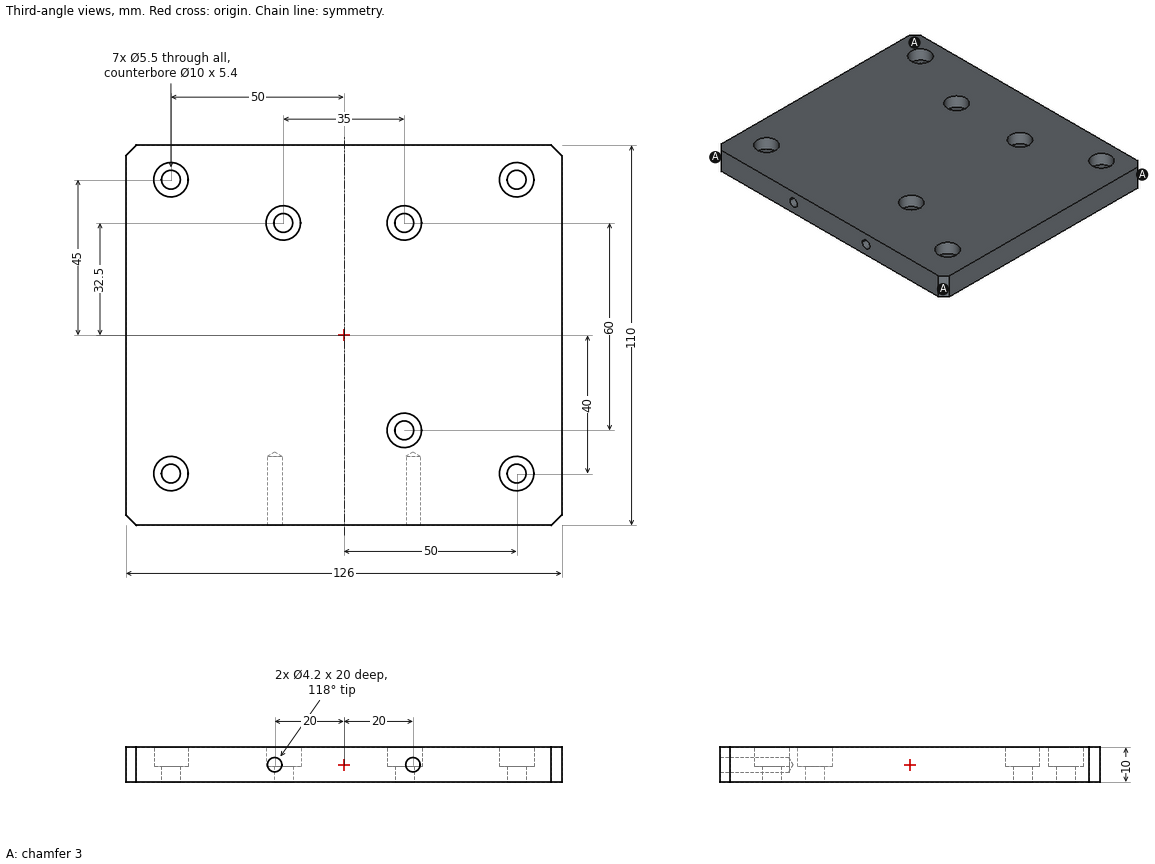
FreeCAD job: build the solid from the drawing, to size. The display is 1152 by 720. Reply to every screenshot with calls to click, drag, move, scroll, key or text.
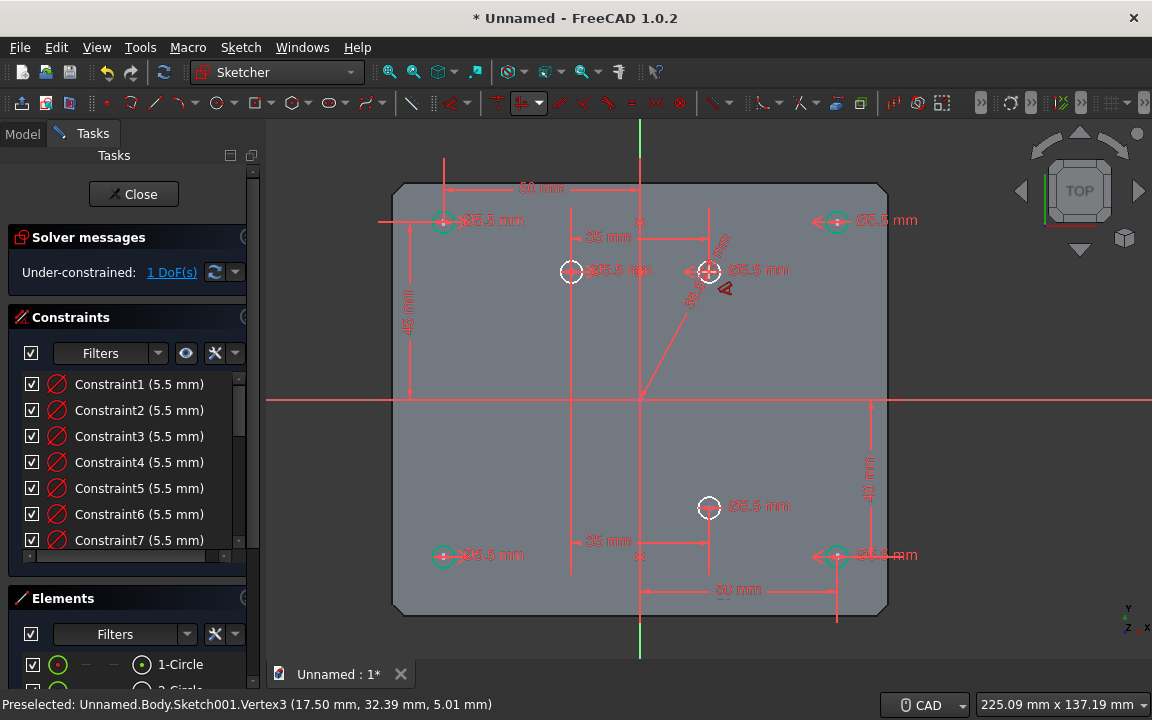
click(709, 508)
click(743, 336)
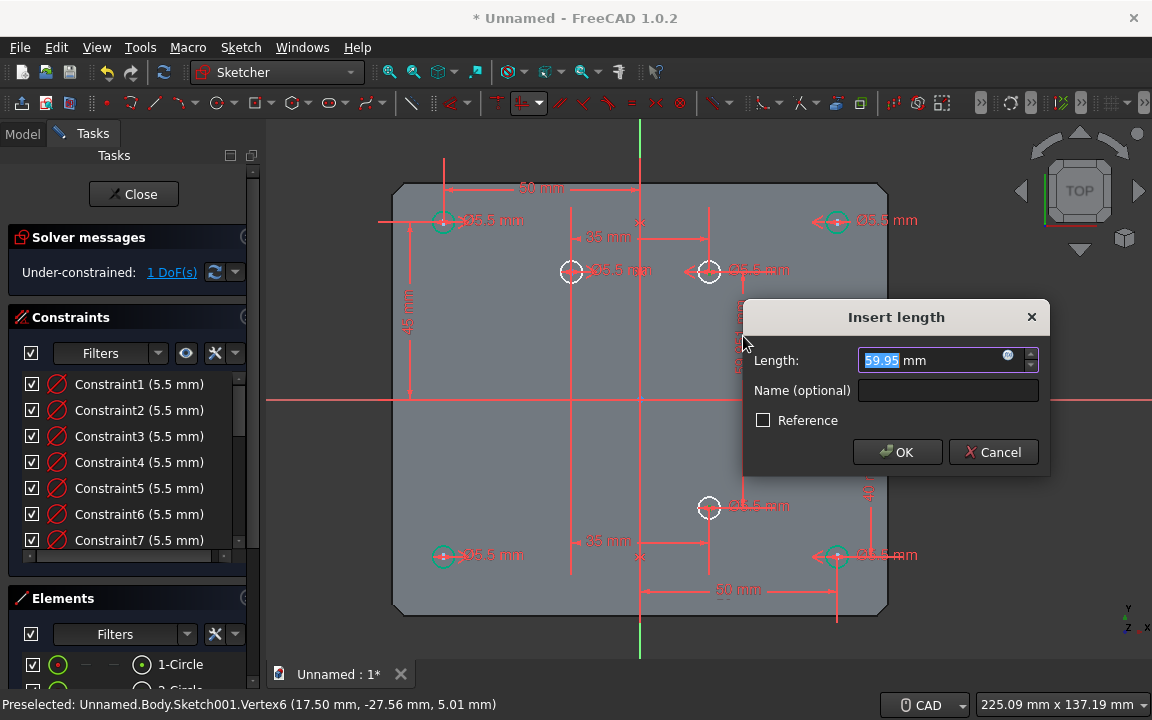
text(60)
key(Return)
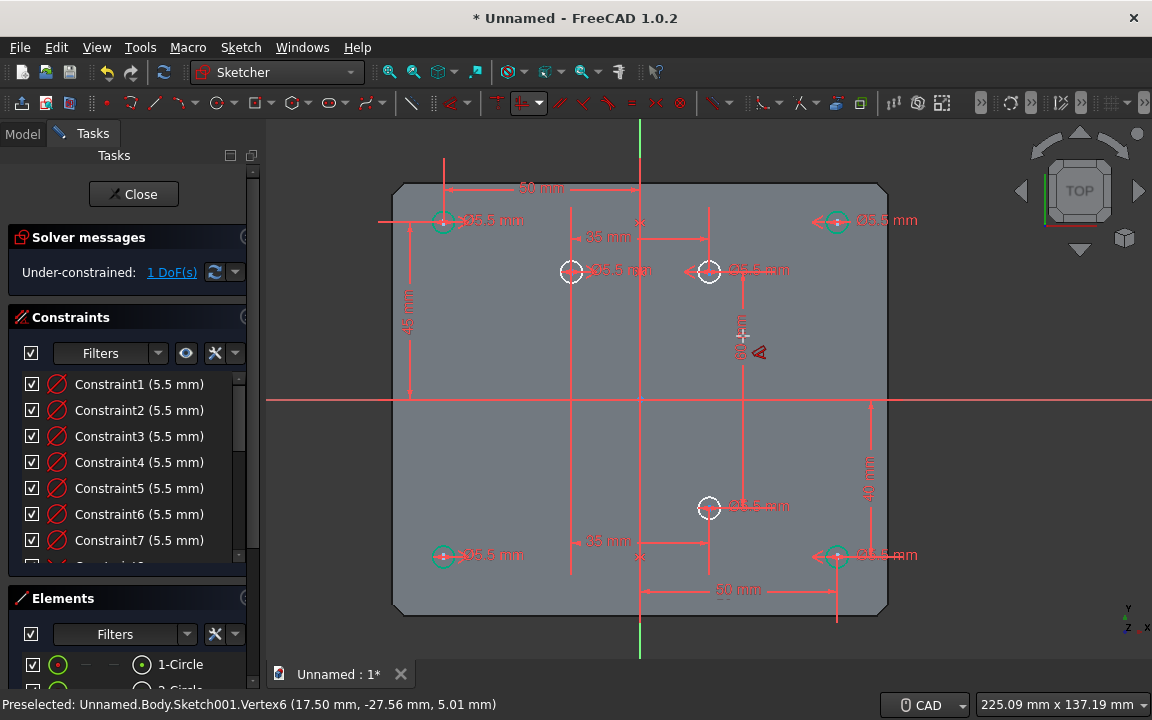
click(571, 272)
click(537, 336)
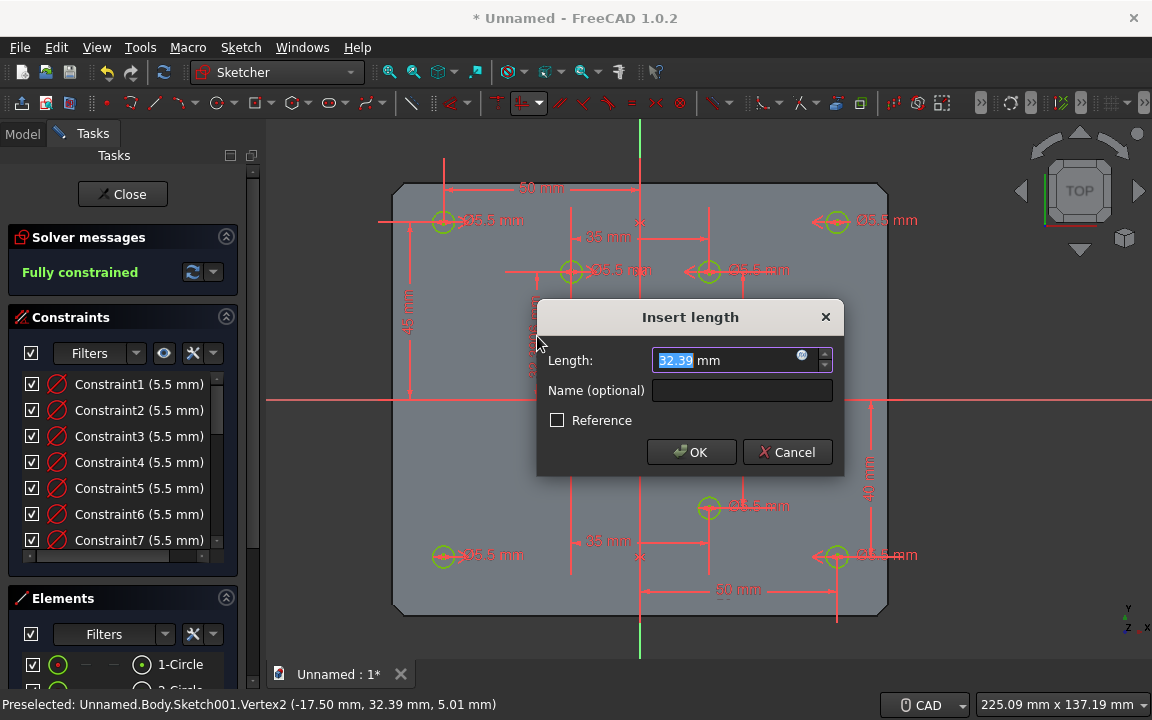
text(32.5)
key(Return)
key(Escape)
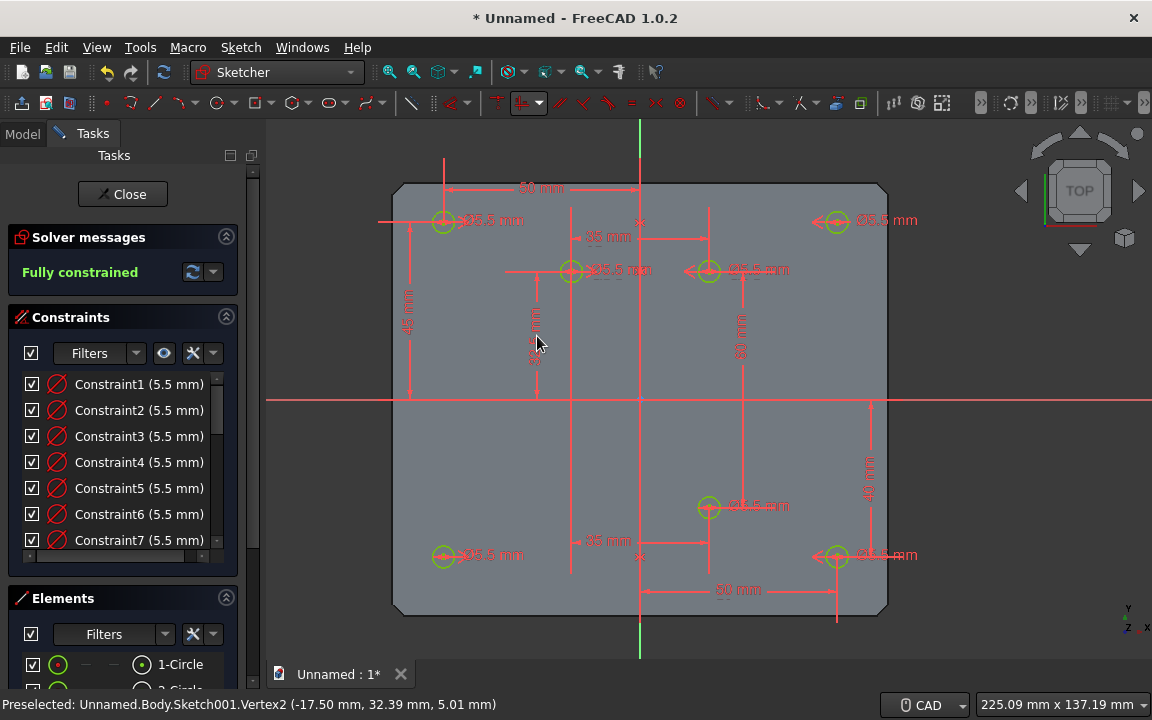
click(123, 194)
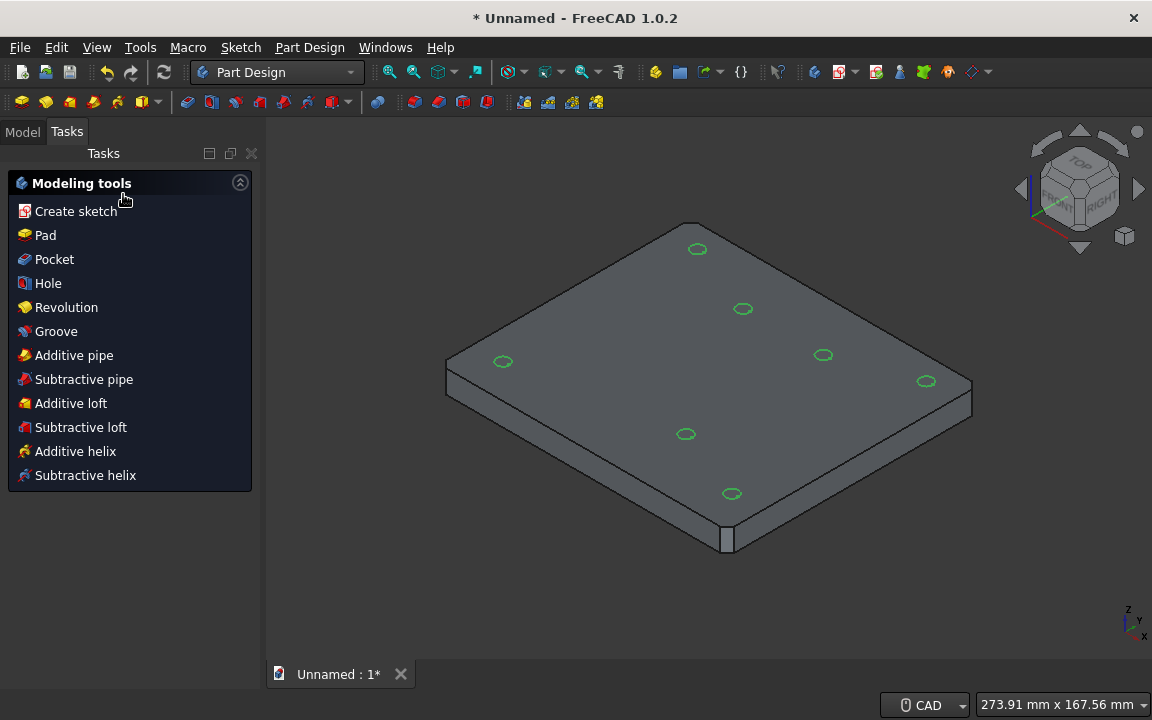
click(212, 102)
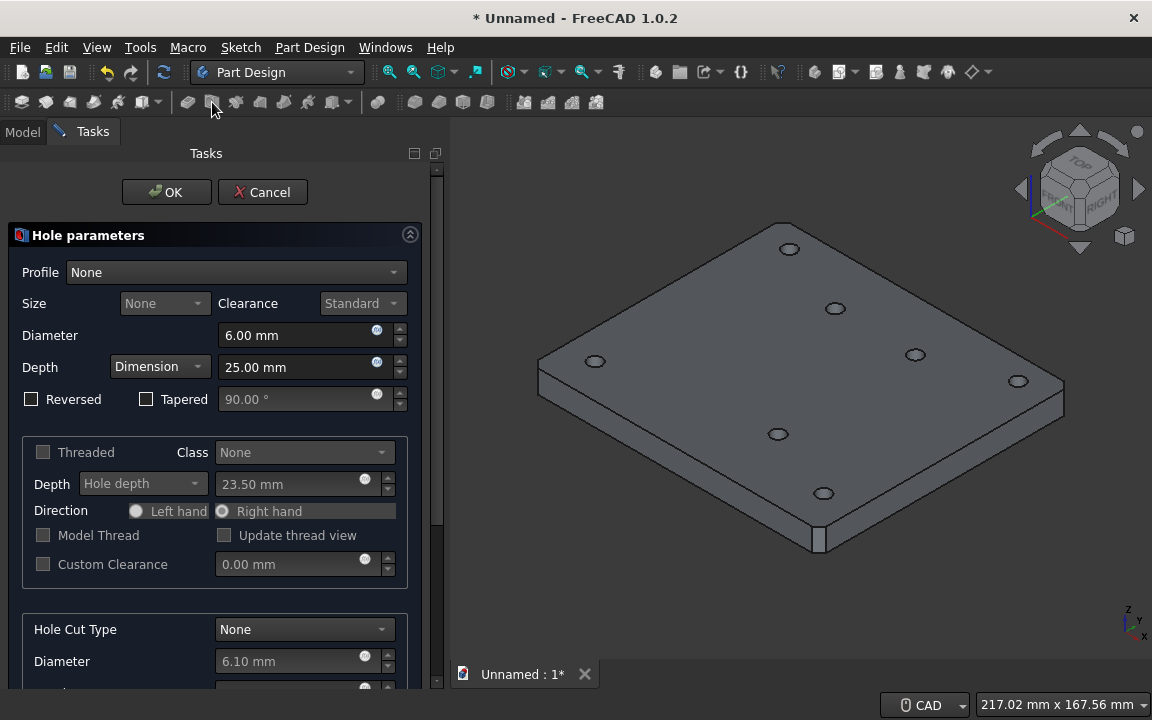
triple_click(305, 335)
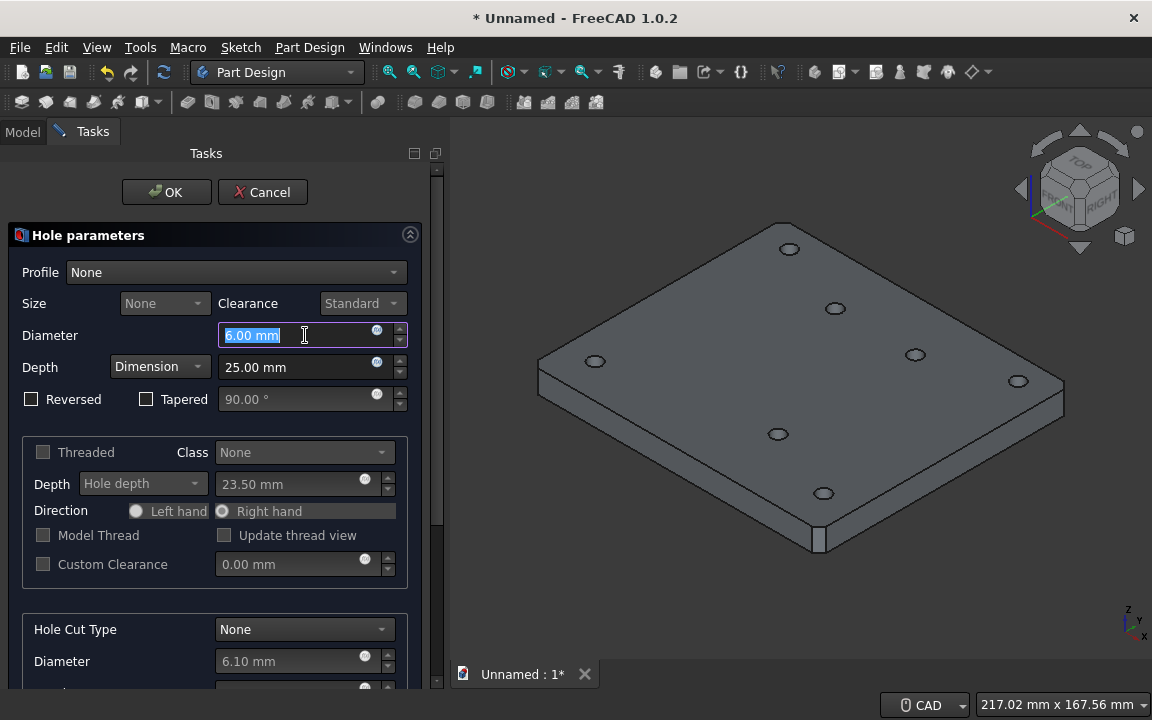
text(5.5)
key(Tab)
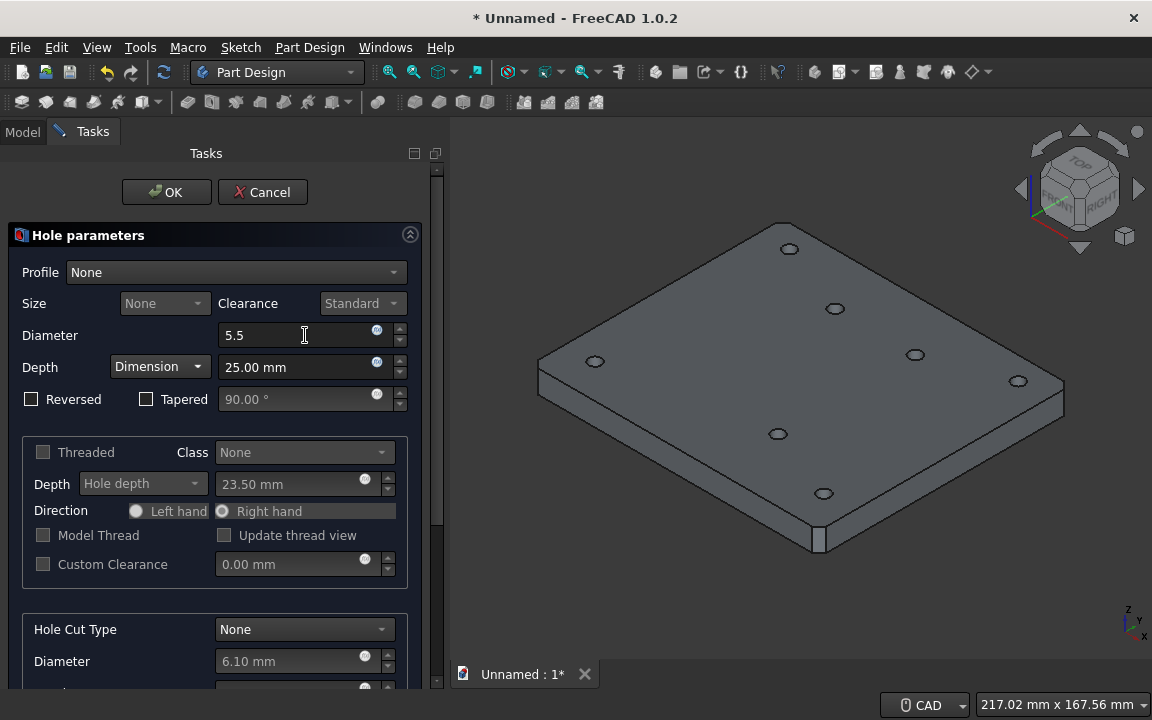
click(161, 366)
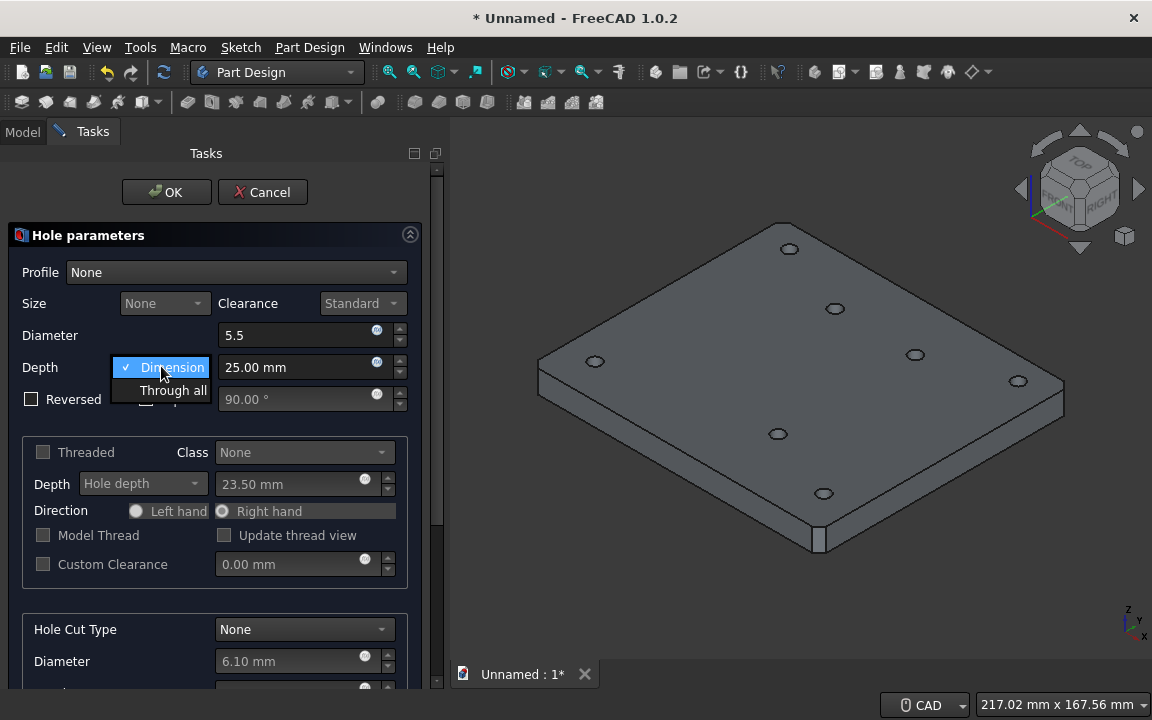
click(160, 390)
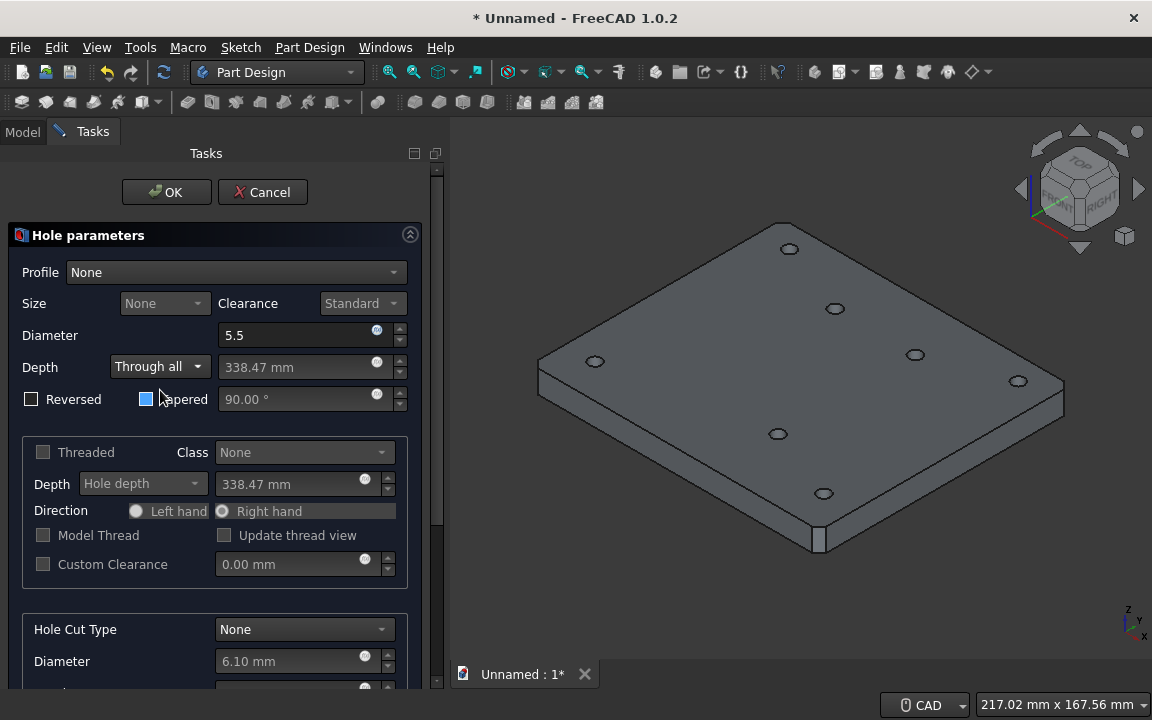
click(306, 630)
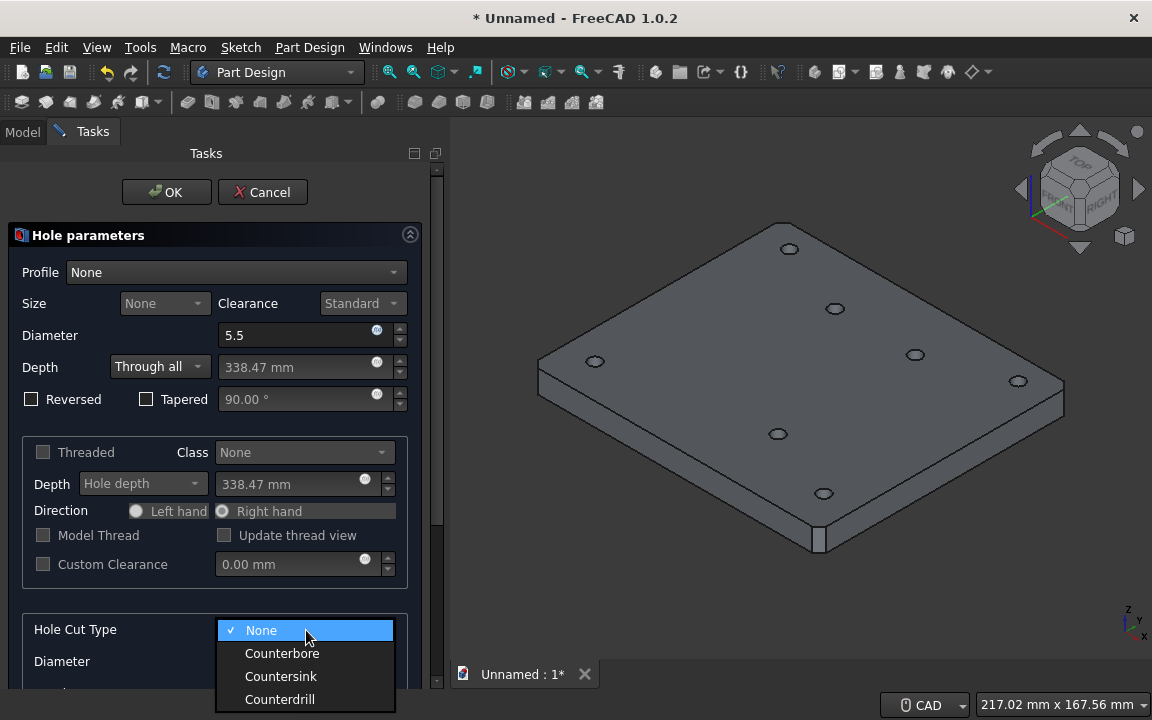
click(304, 654)